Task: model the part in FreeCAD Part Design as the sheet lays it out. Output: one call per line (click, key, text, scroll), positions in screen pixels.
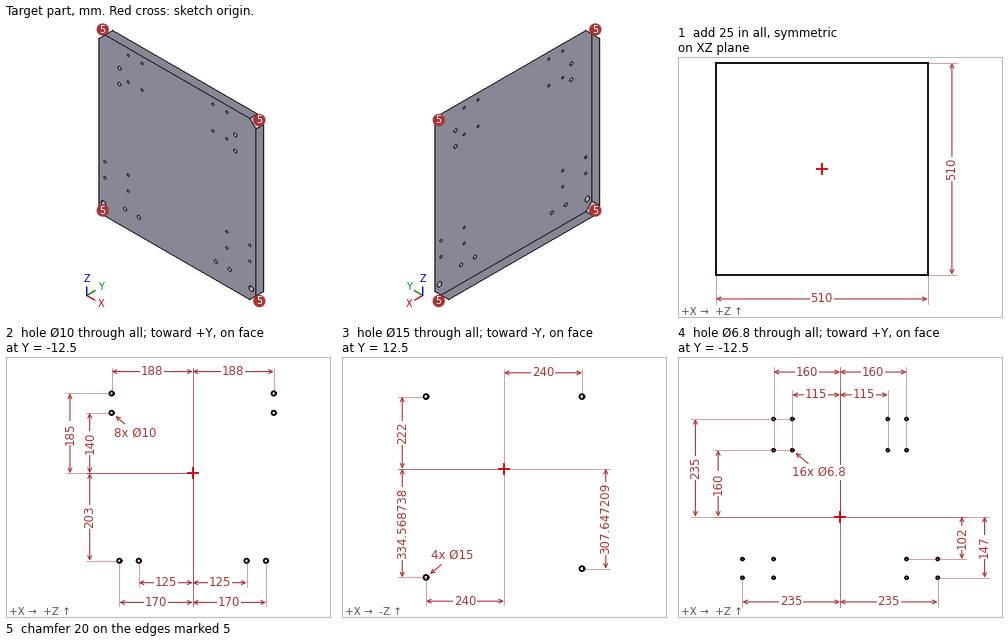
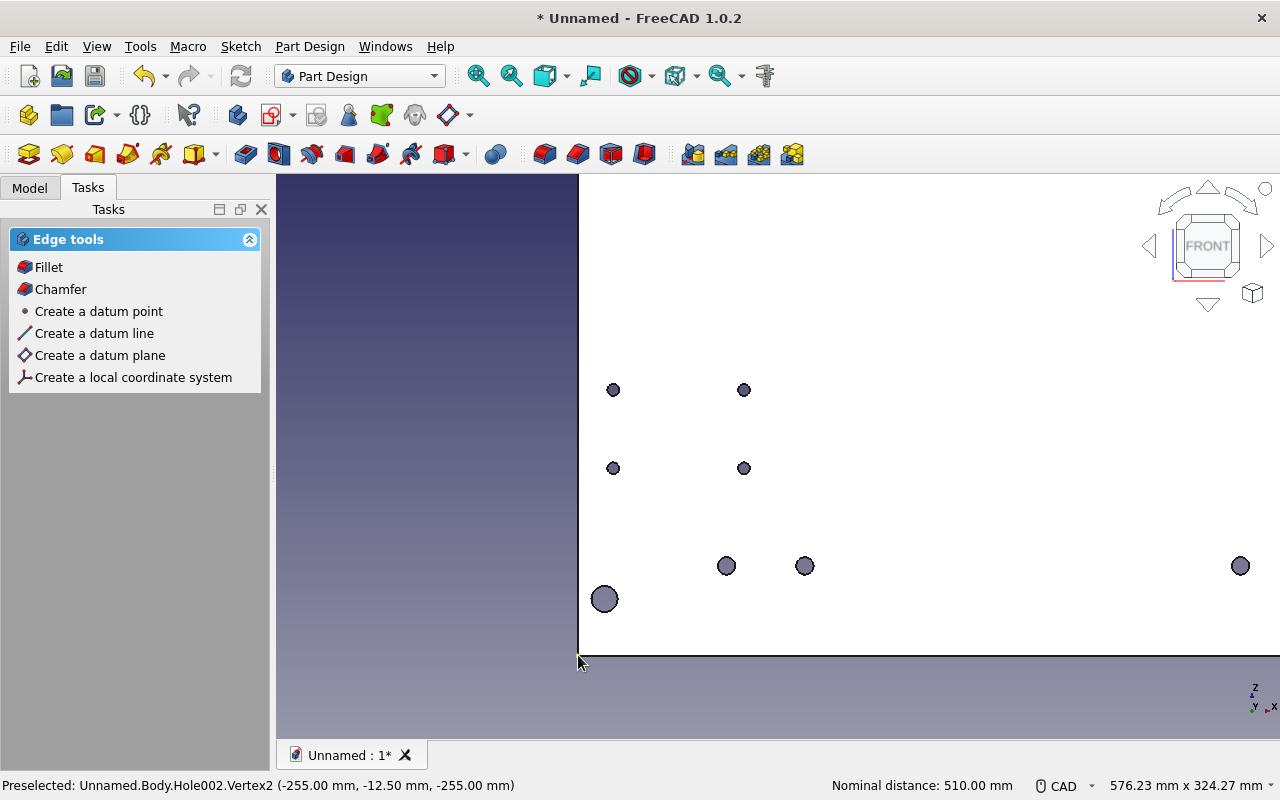
click(479, 76)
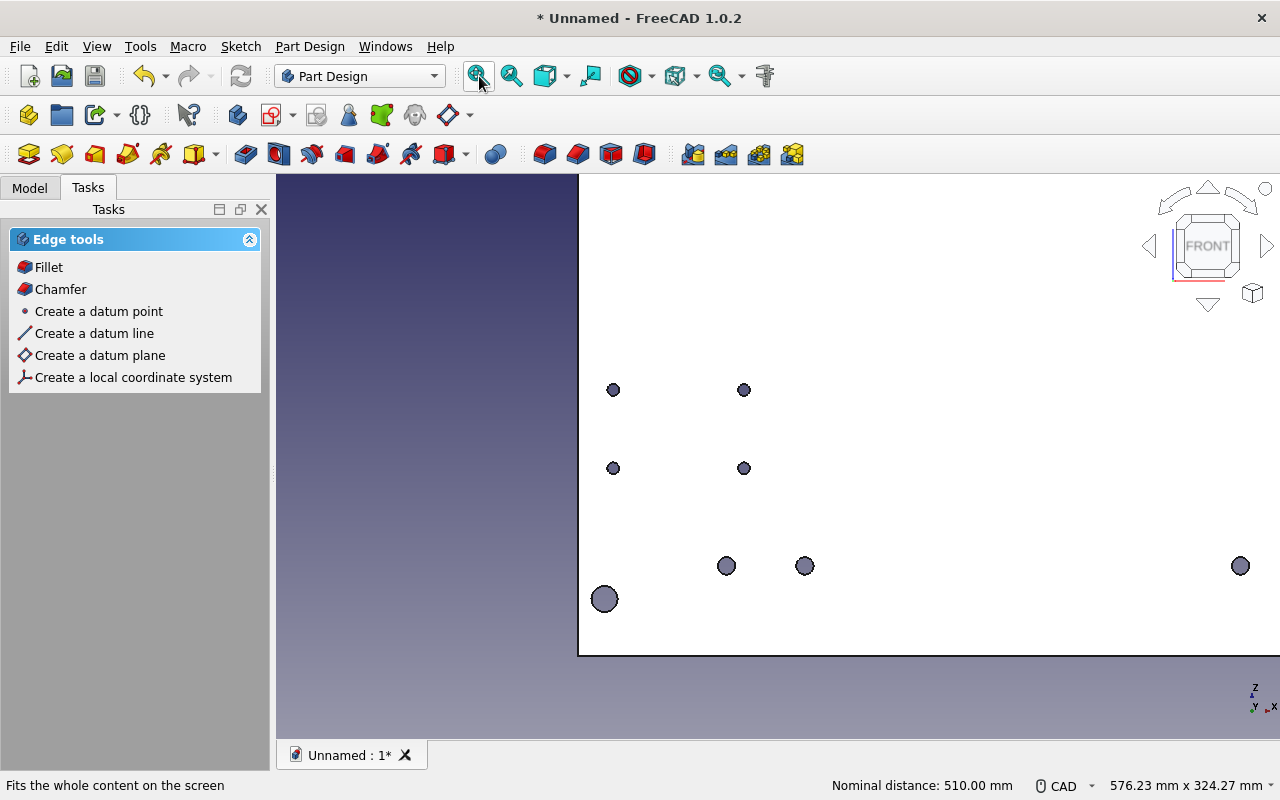
key(3)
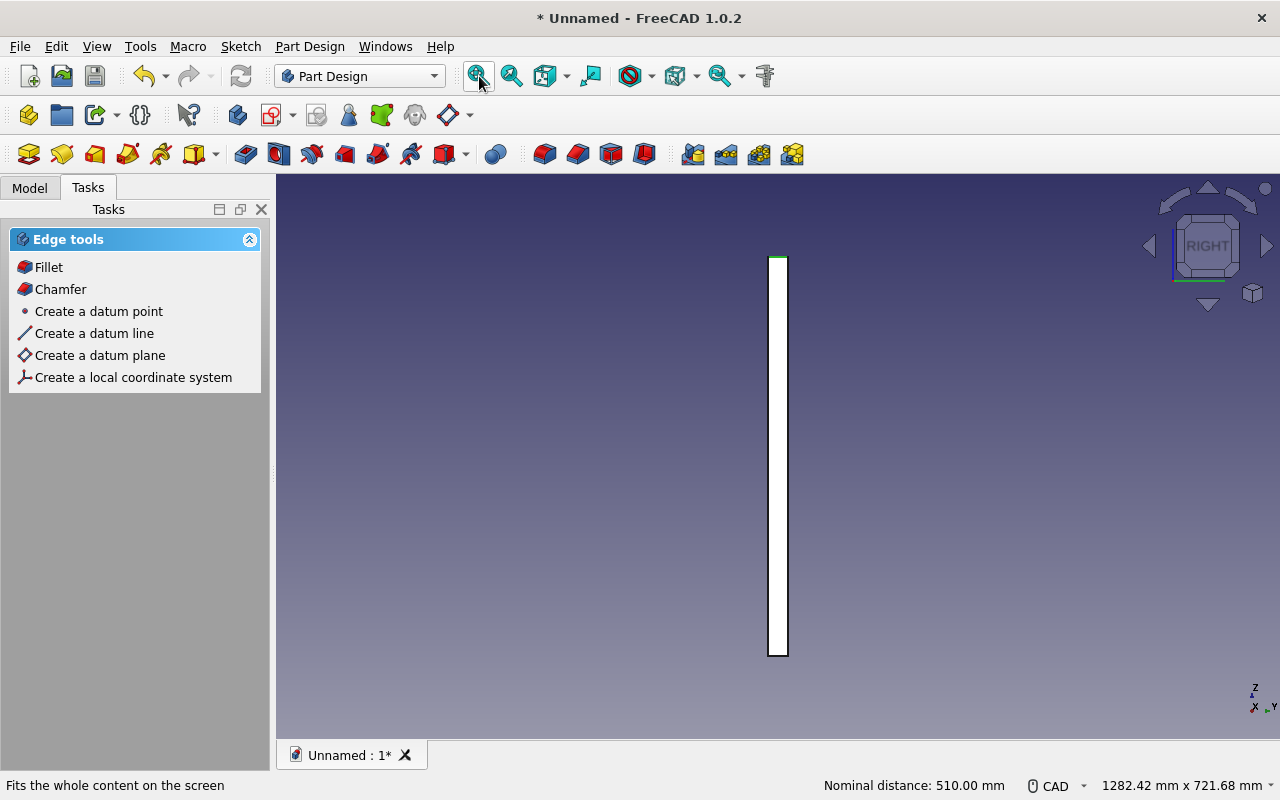
click(778, 655, ctrl)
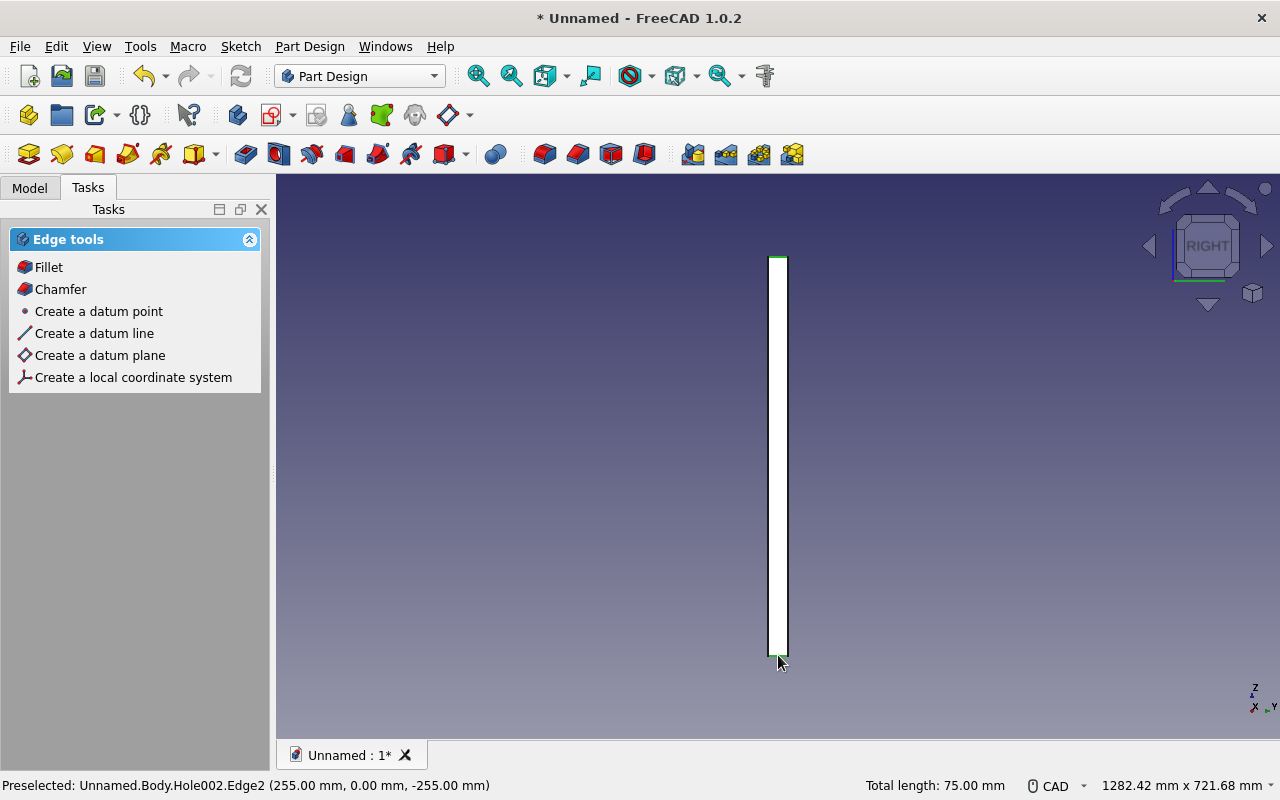
scroll(778, 655, up, 4)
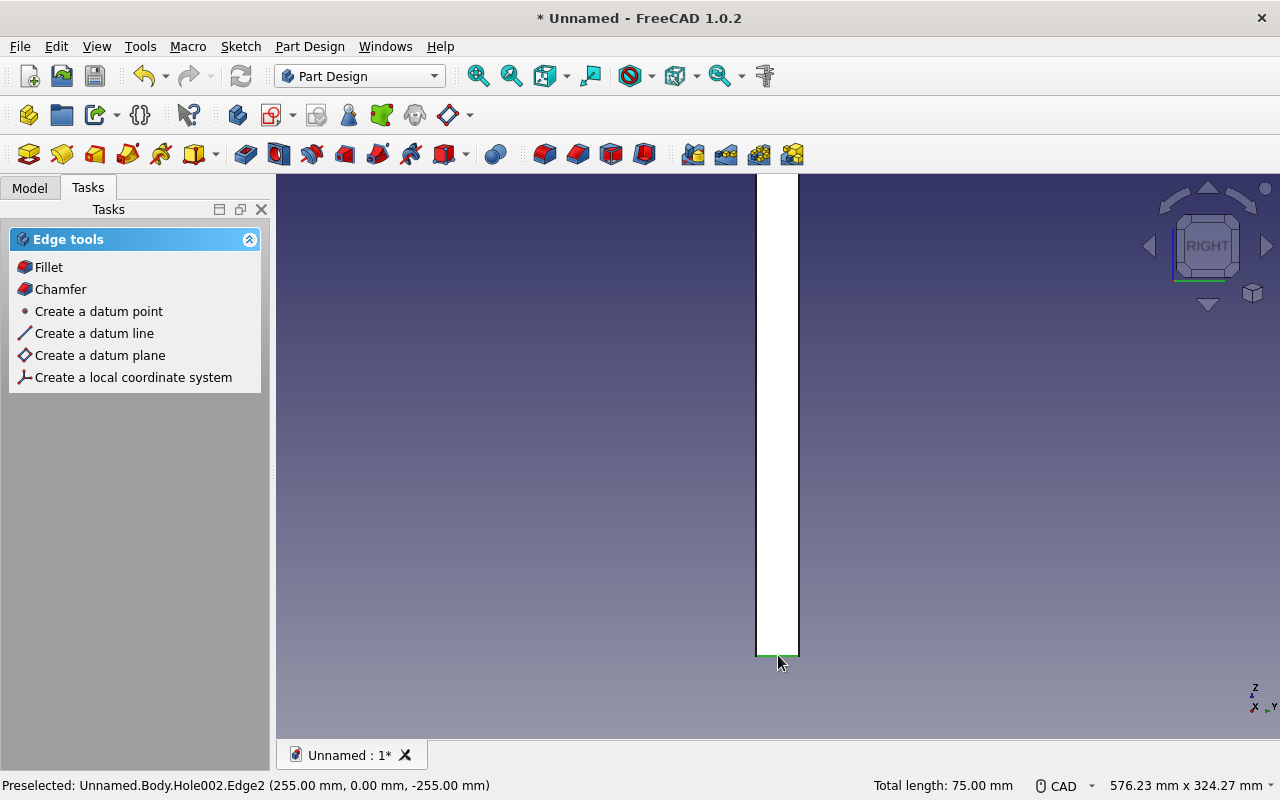
key(v)
key(f)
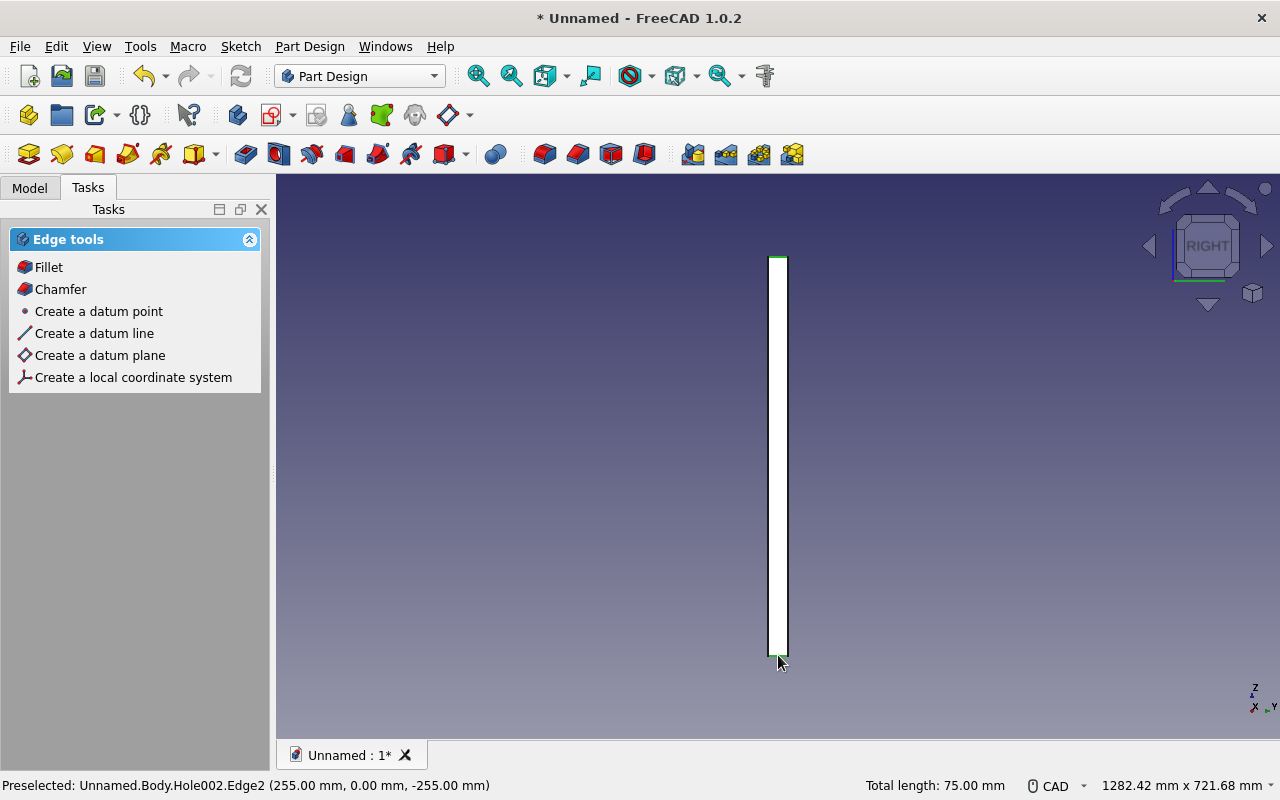
key(5)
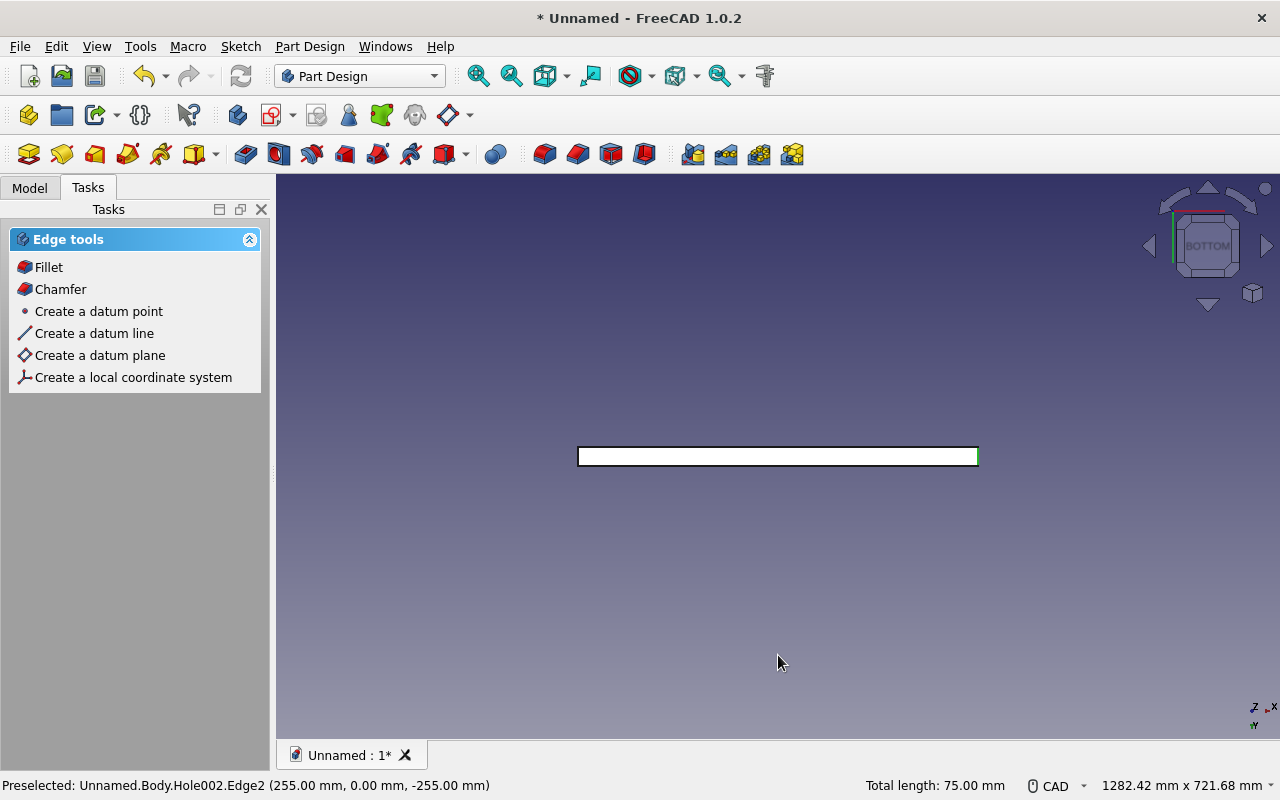
click(479, 76)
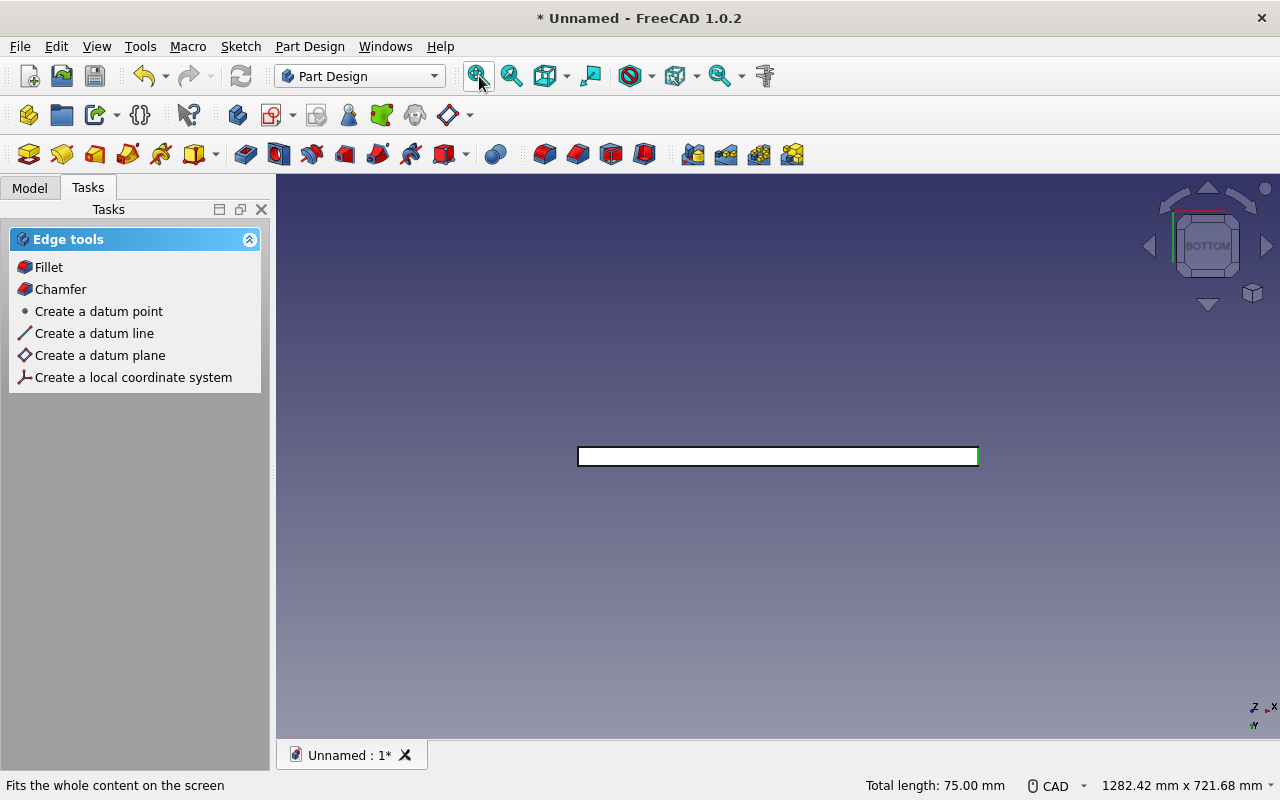
click(578, 455, ctrl)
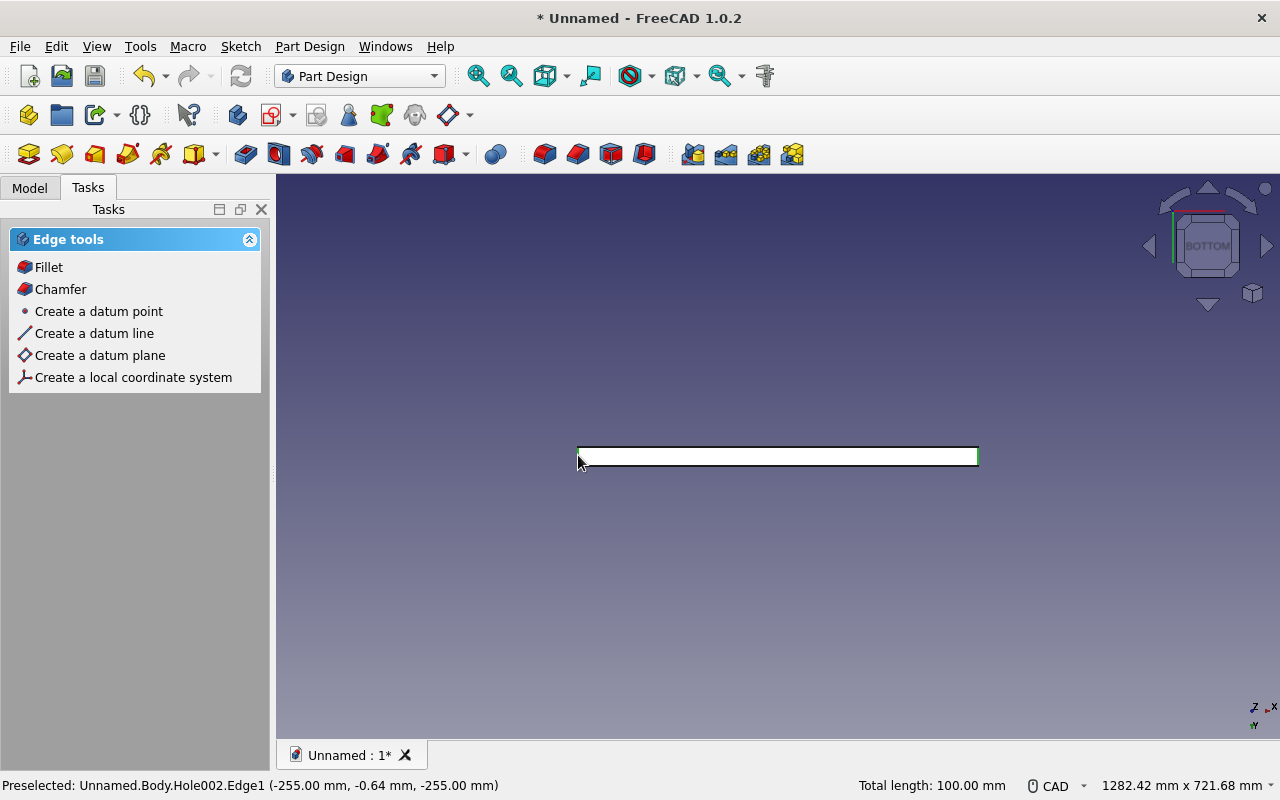
click(578, 154)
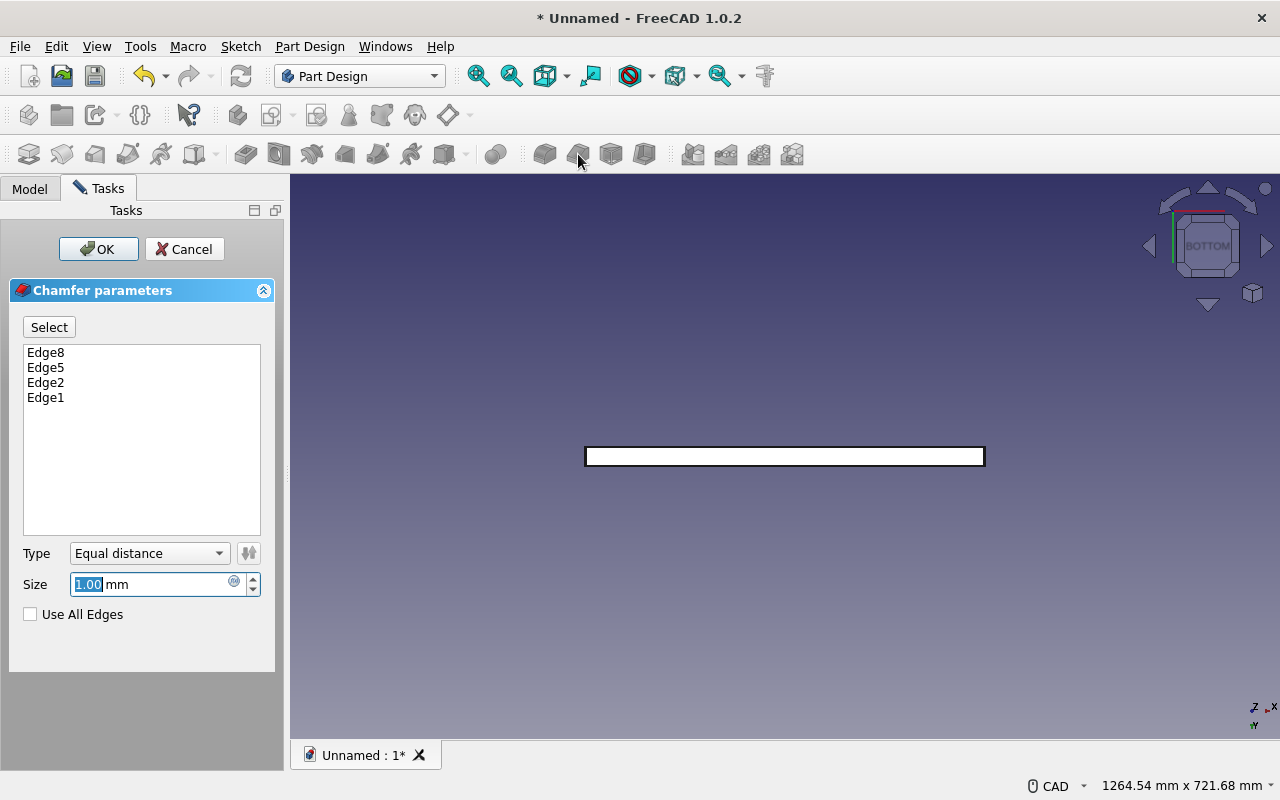
text(20)
key(Tab)